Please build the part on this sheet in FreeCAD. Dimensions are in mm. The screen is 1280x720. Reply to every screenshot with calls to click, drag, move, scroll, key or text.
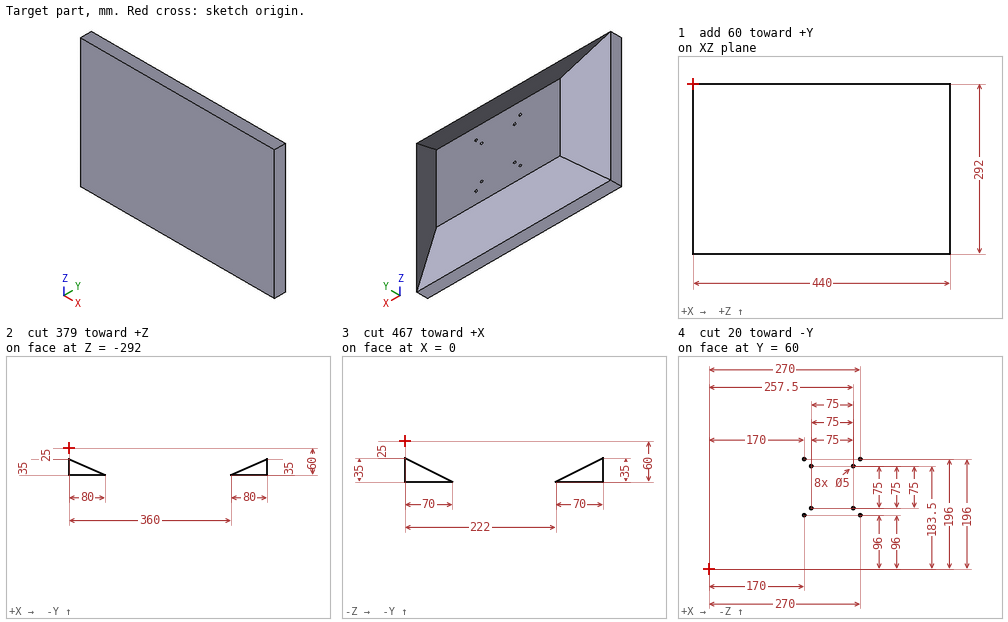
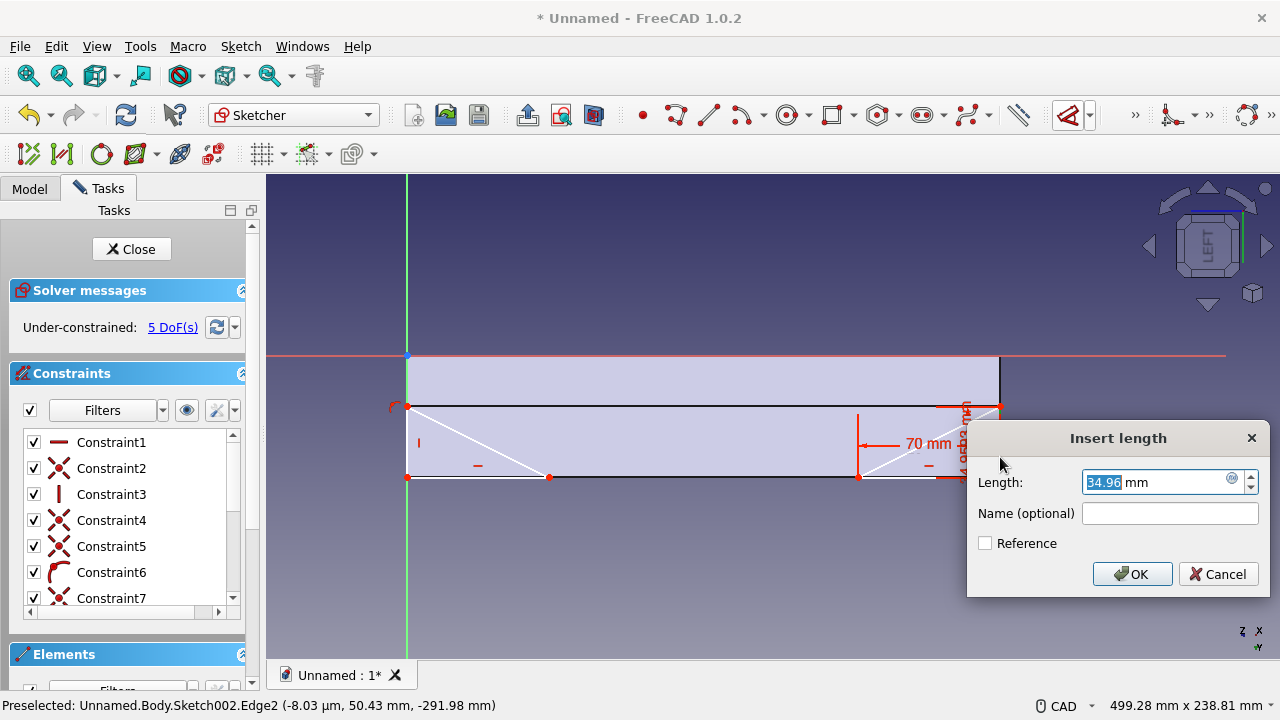
text(35)
key(Return)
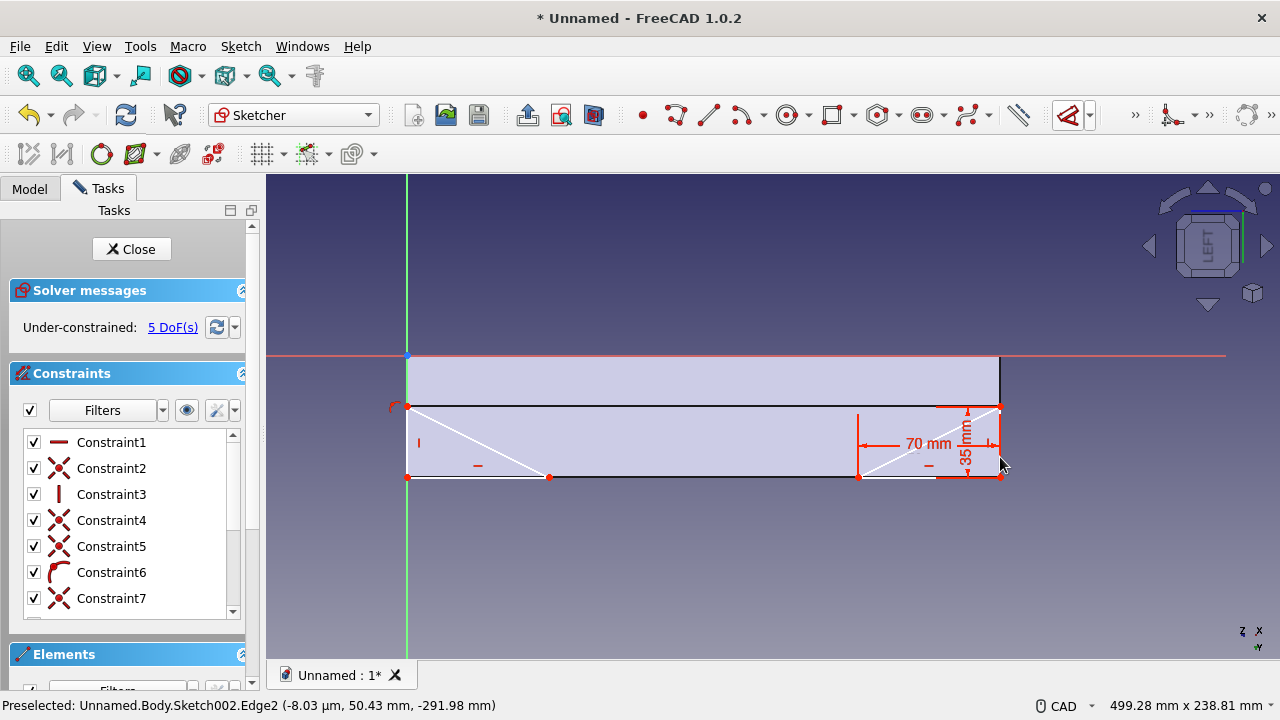
click(407, 428)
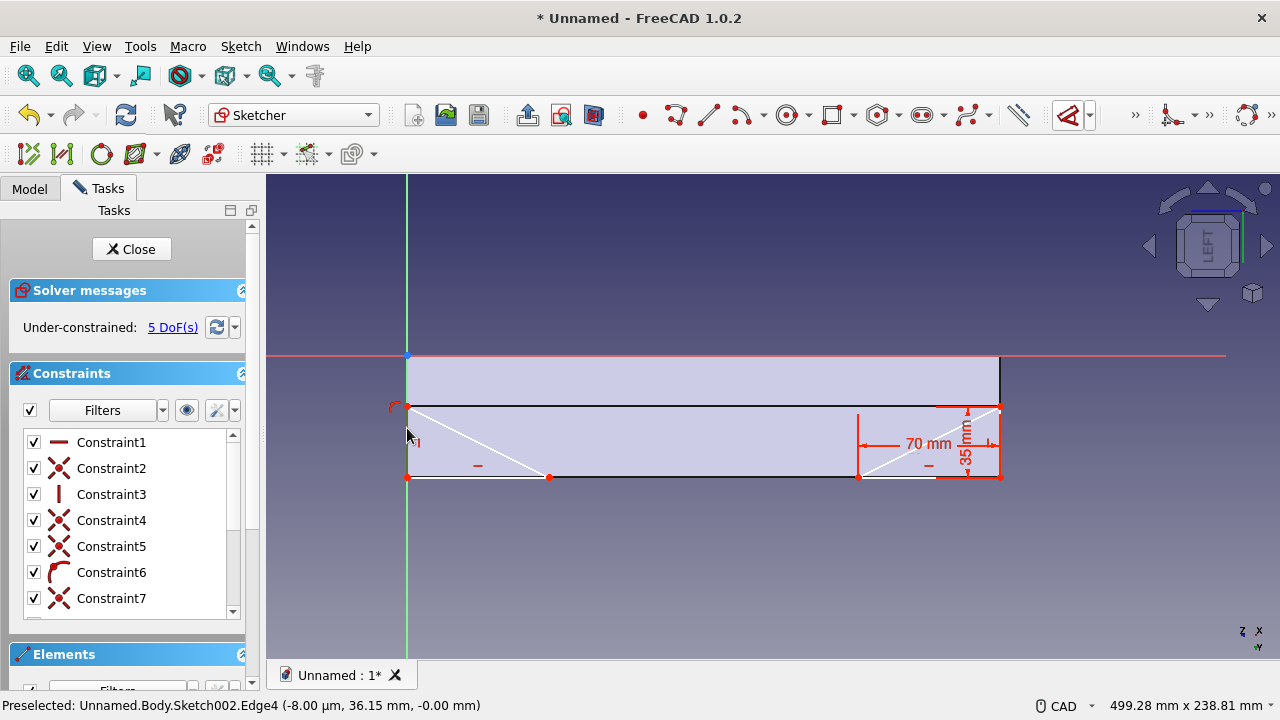
click(1090, 116)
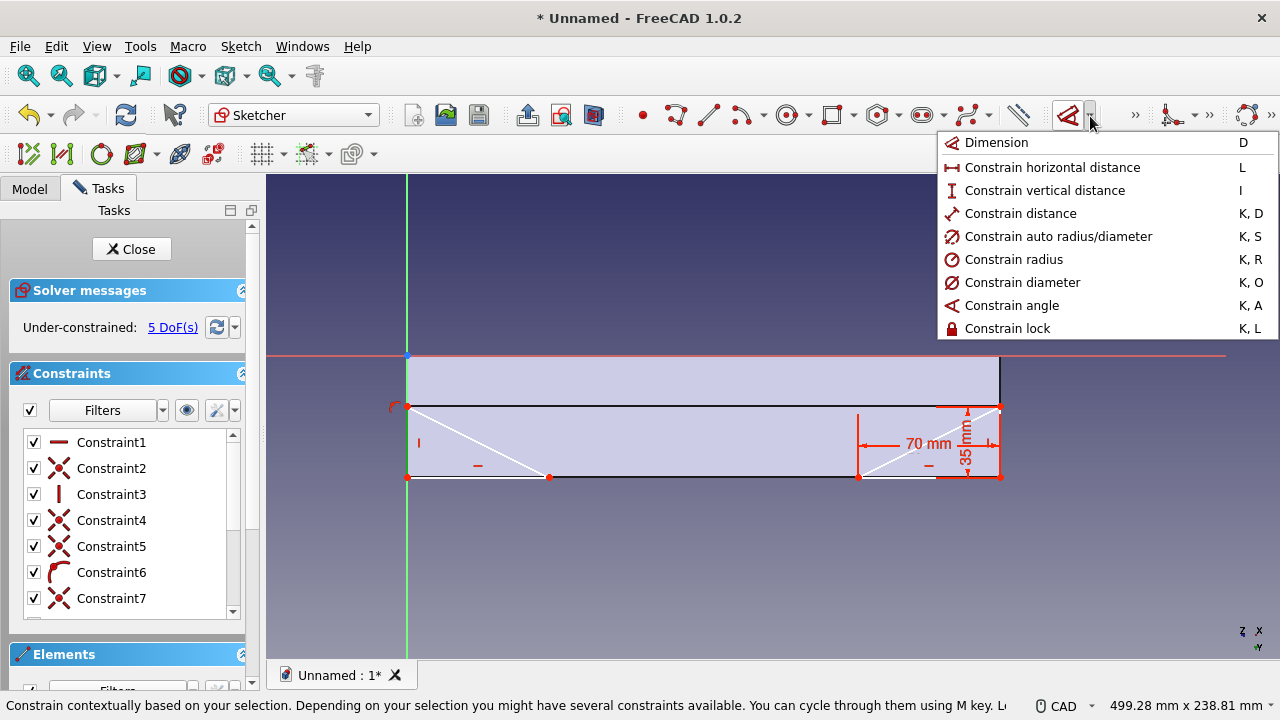
click(1108, 190)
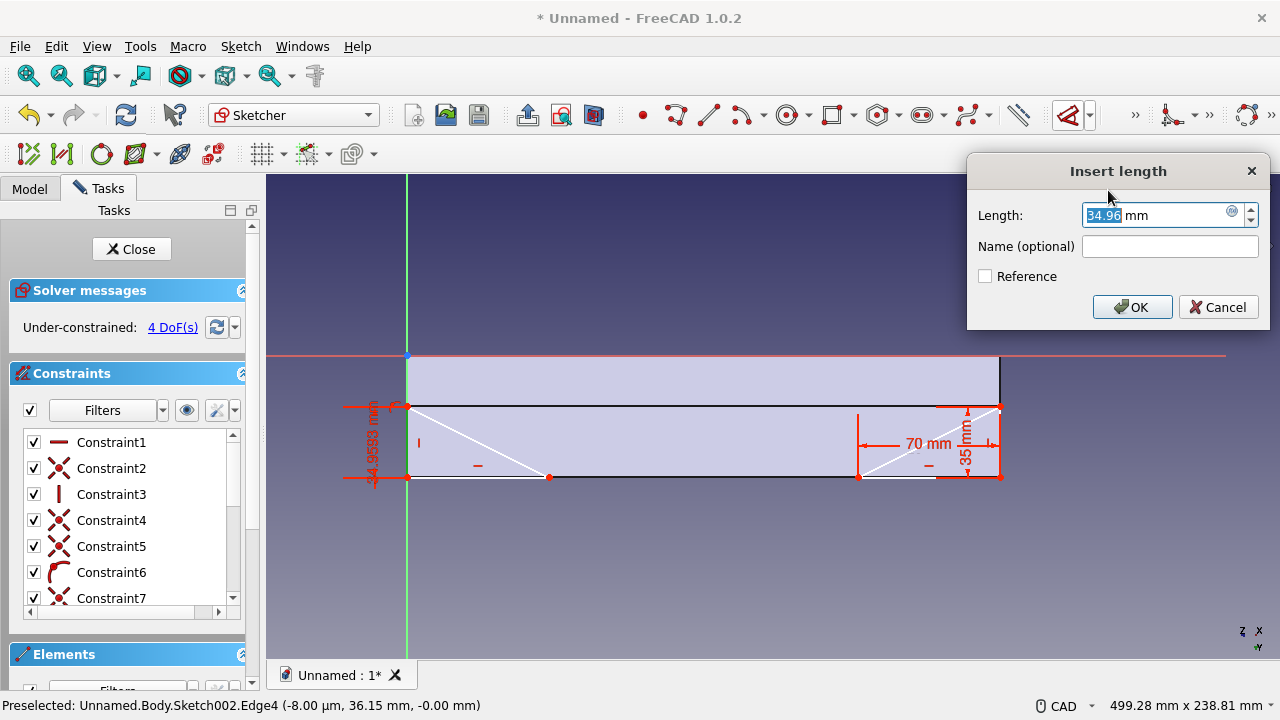
text(35)
key(Return)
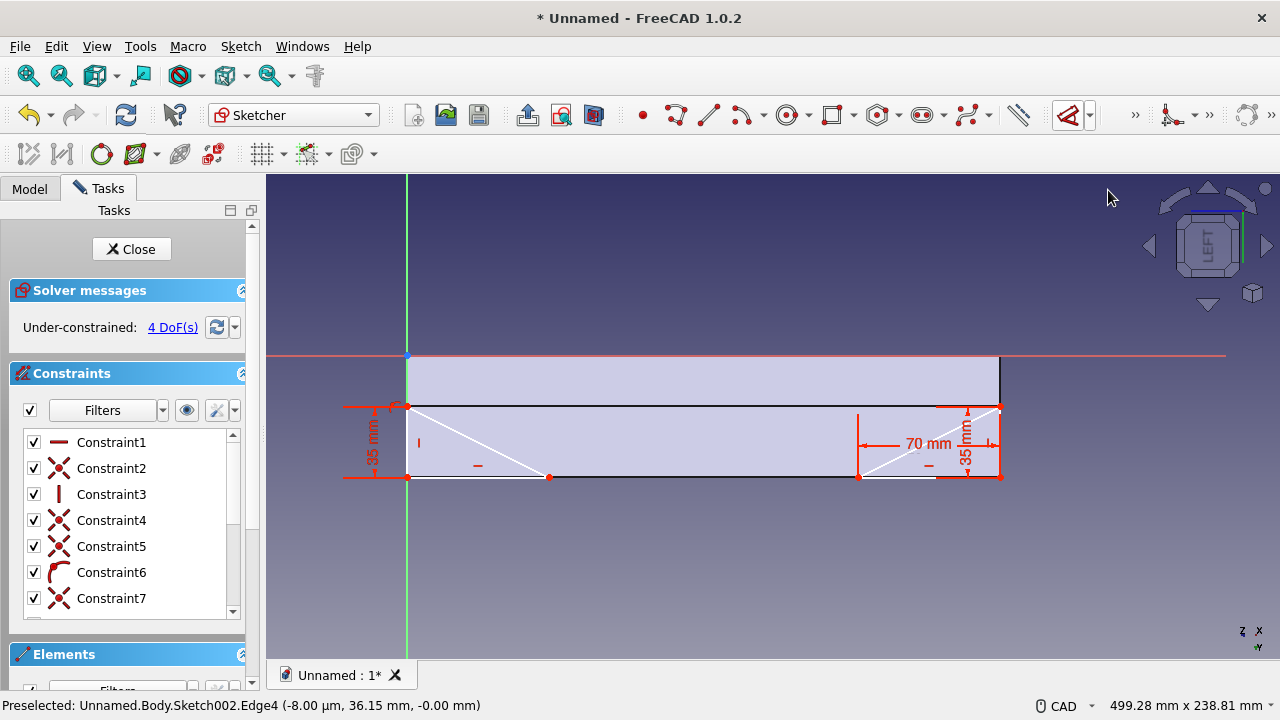
click(450, 478)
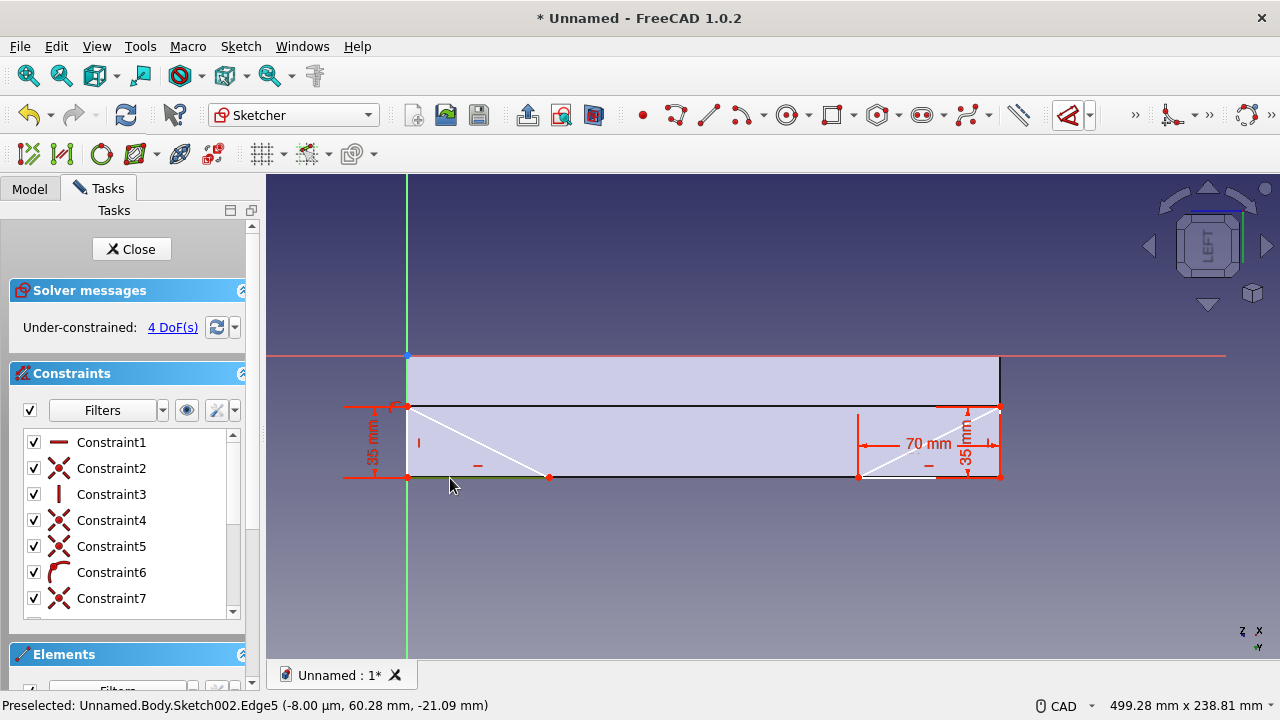
key(l)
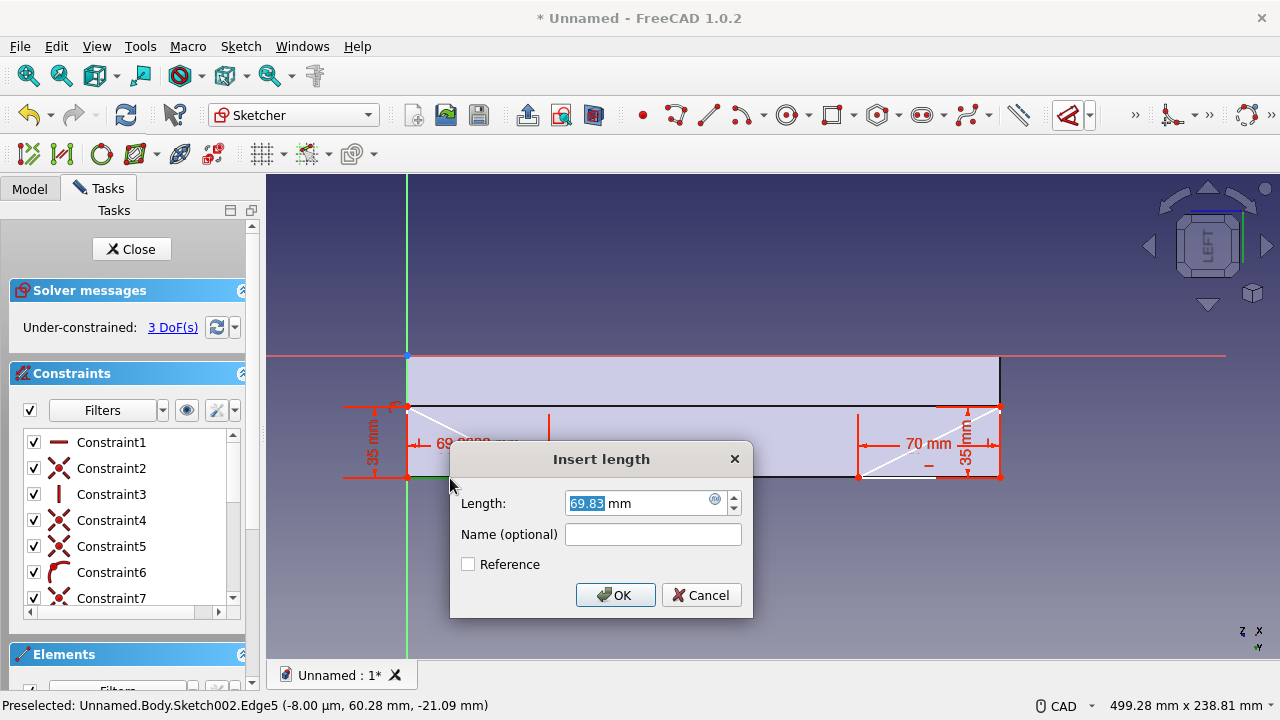
text(70)
key(Return)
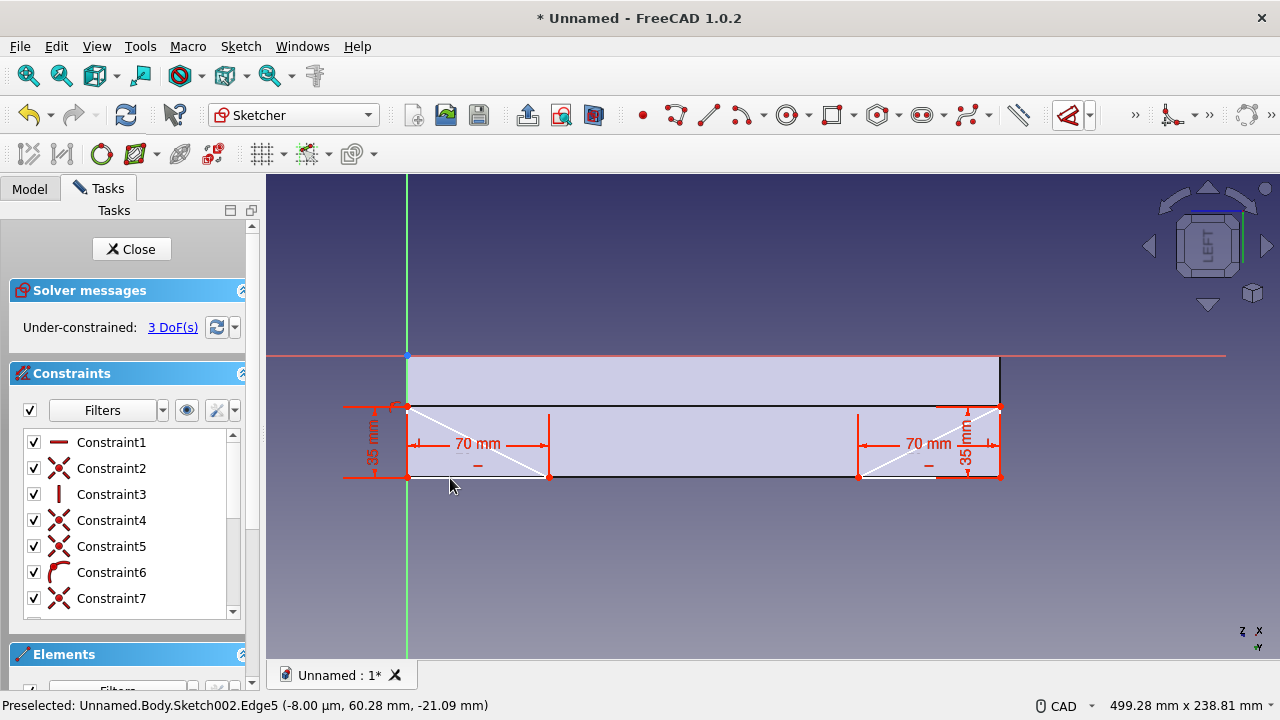
click(858, 478)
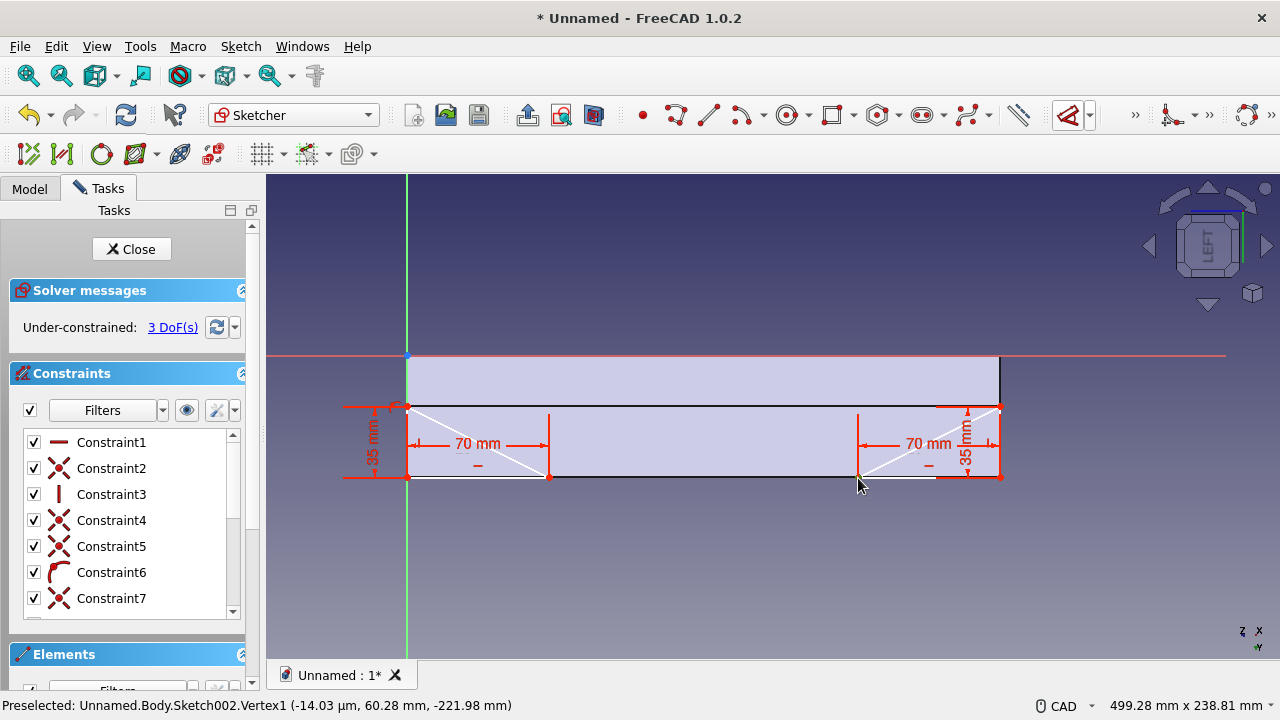
key(i)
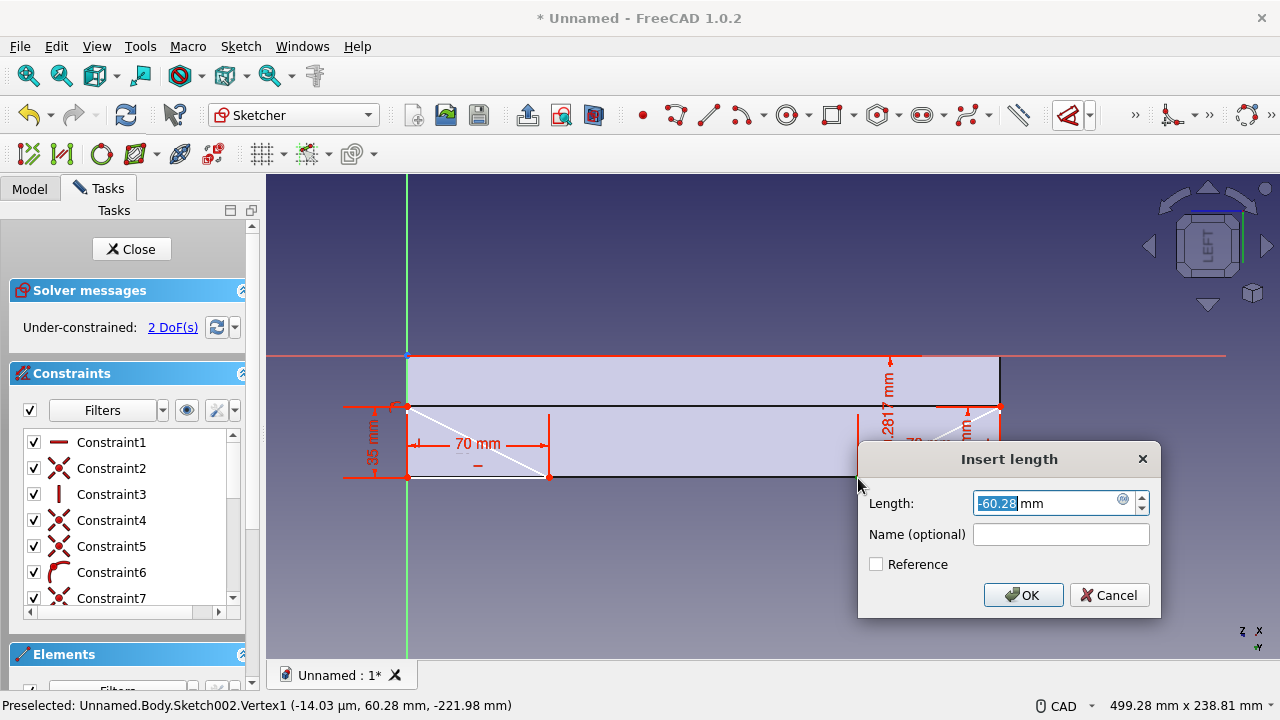
text(-60)
key(Return)